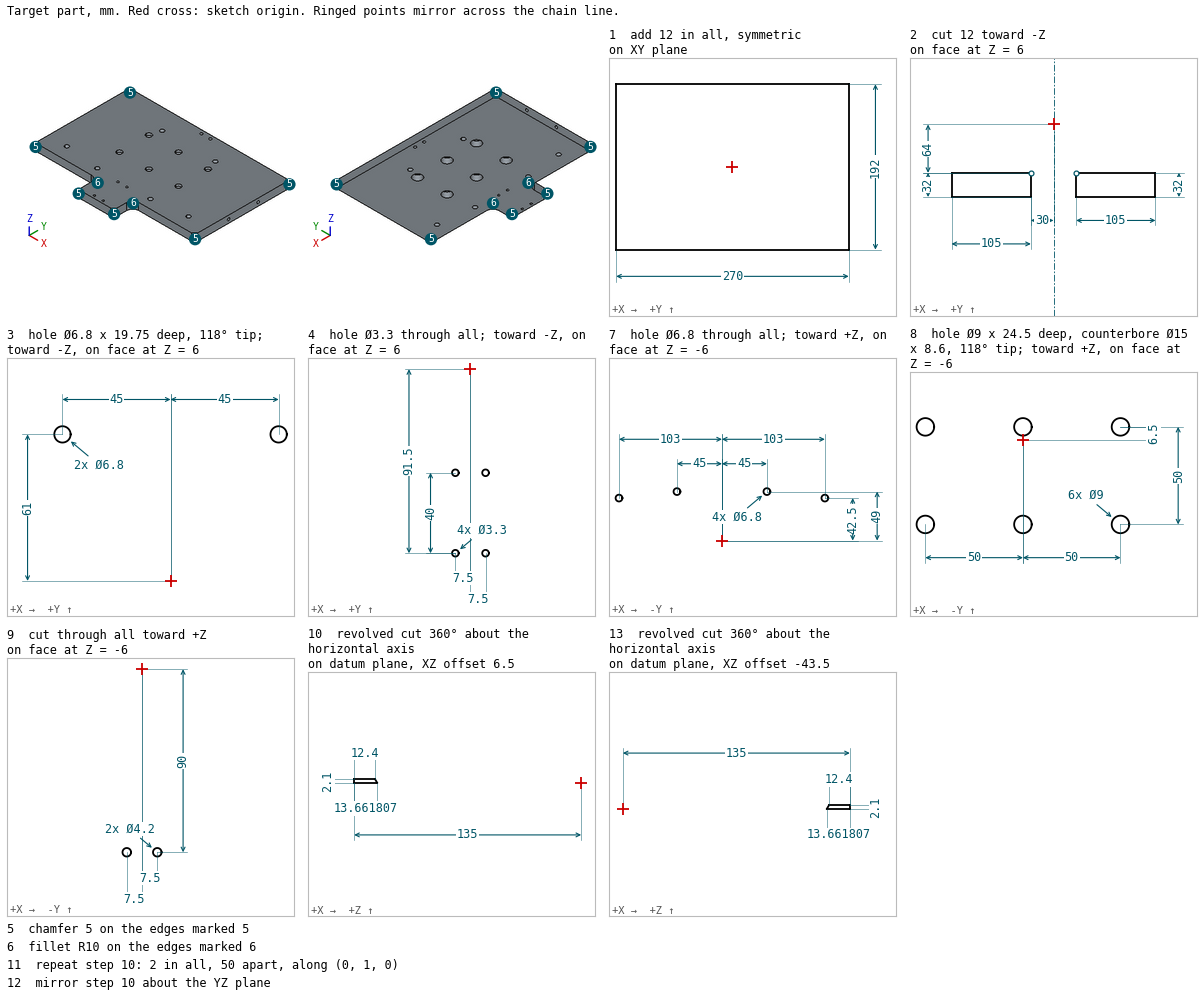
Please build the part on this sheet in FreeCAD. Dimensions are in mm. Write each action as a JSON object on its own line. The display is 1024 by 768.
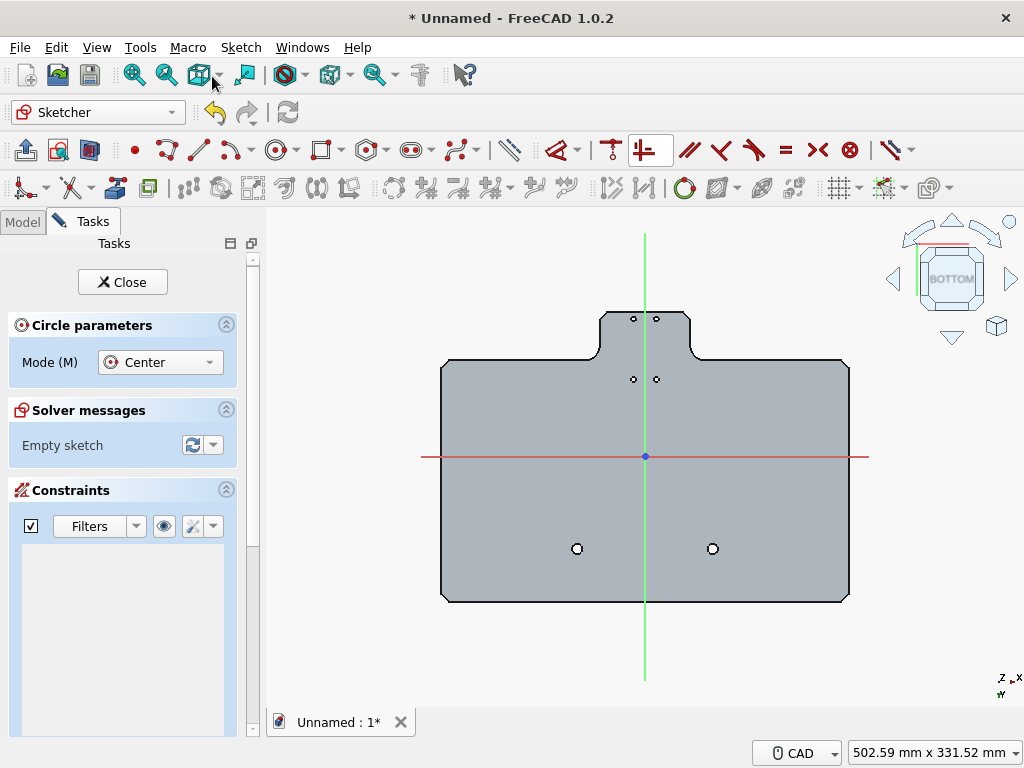
{"action": "scroll", "coordinate": [713, 383], "scroll_direction": "up", "scroll_amount": 8}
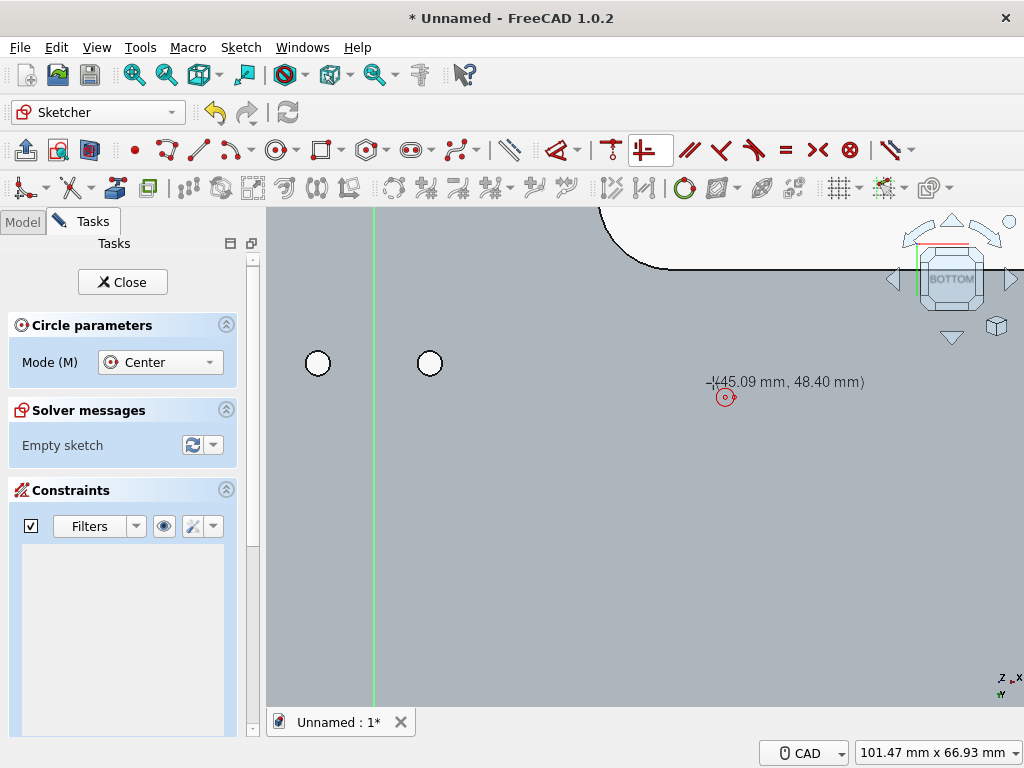
{"action": "scroll", "coordinate": [643, 426], "scroll_direction": "down", "scroll_amount": 7}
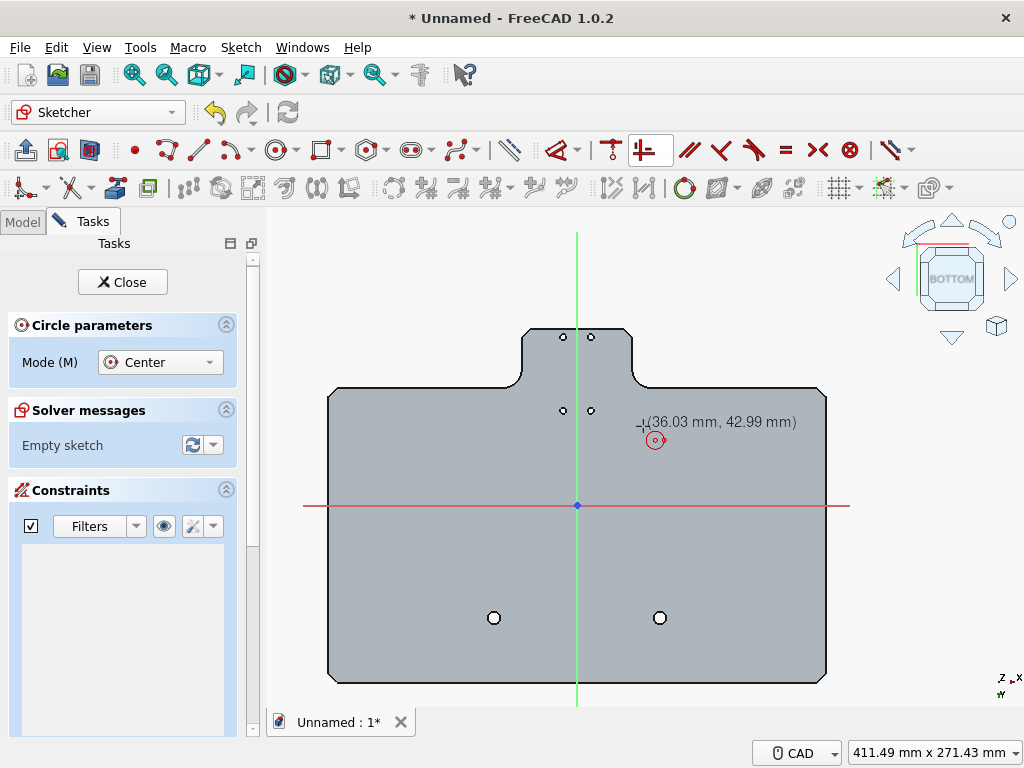
{"action": "left_click", "coordinate": [660, 416]}
{"action": "mouse_move", "coordinate": [664, 411]}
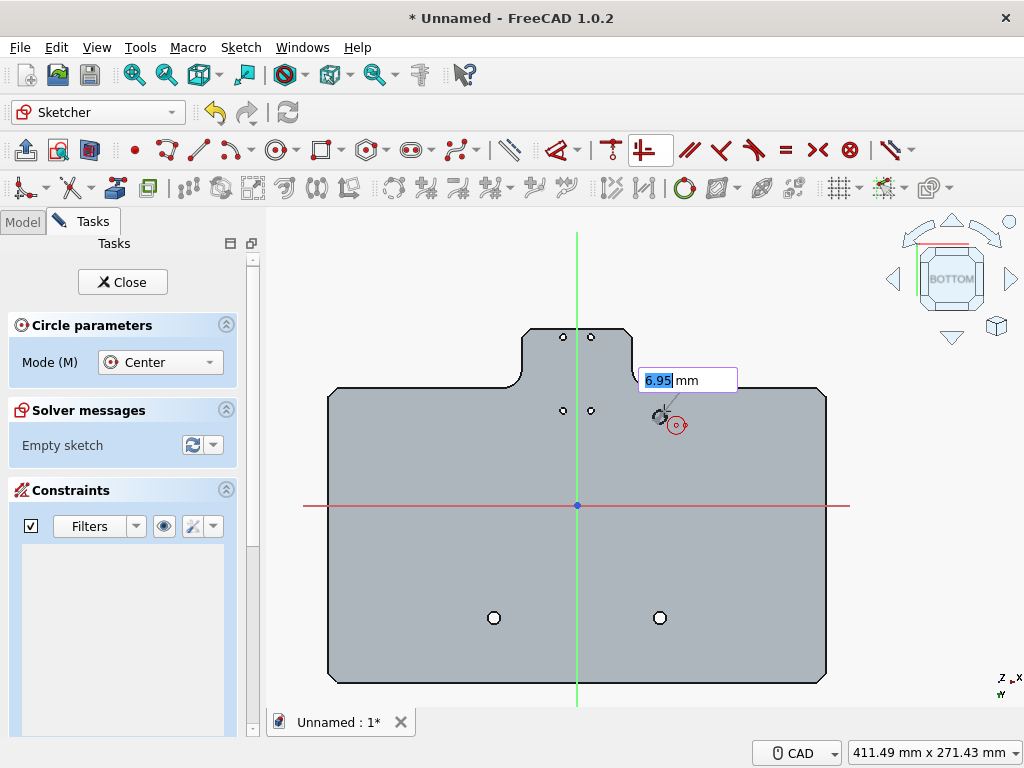
{"action": "type", "text": "6.8"}
{"action": "key", "text": "Return"}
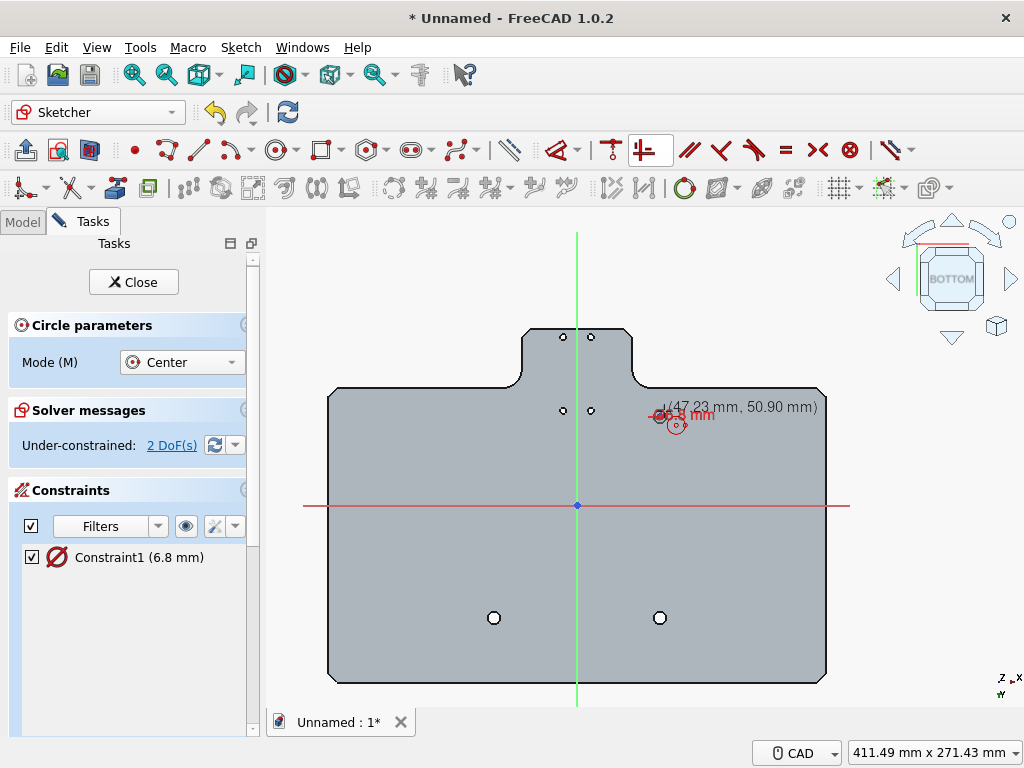
{"action": "scroll", "coordinate": [494, 416], "scroll_direction": "up", "scroll_amount": 7}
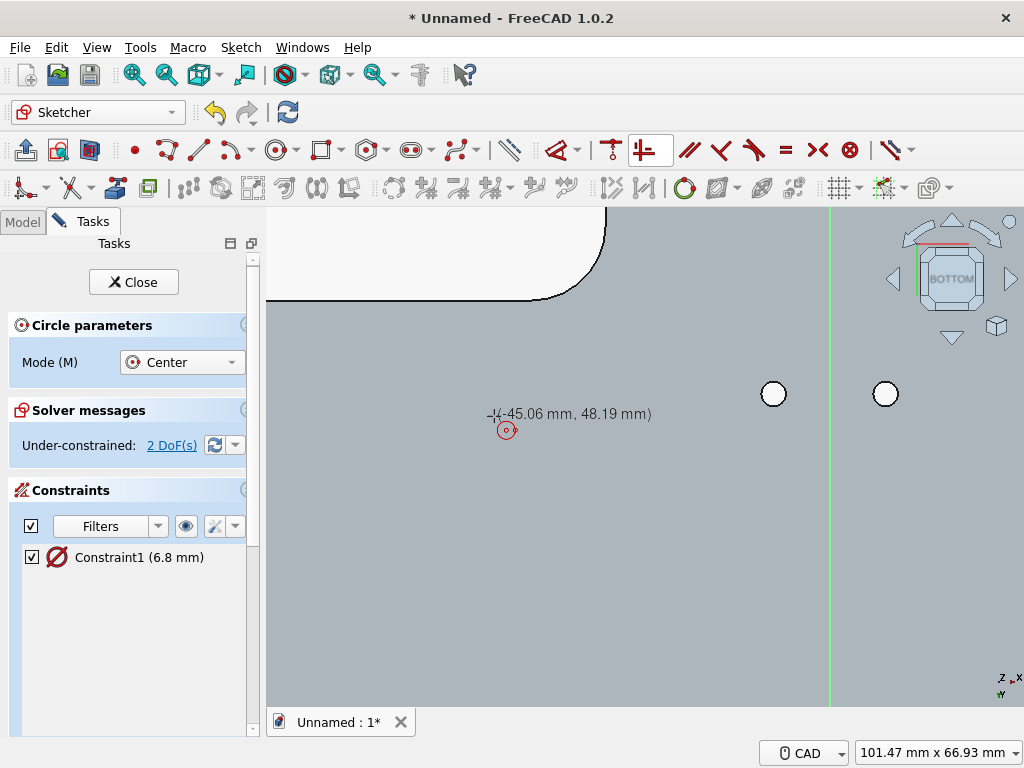
{"action": "scroll", "coordinate": [494, 416], "scroll_direction": "down", "scroll_amount": 7}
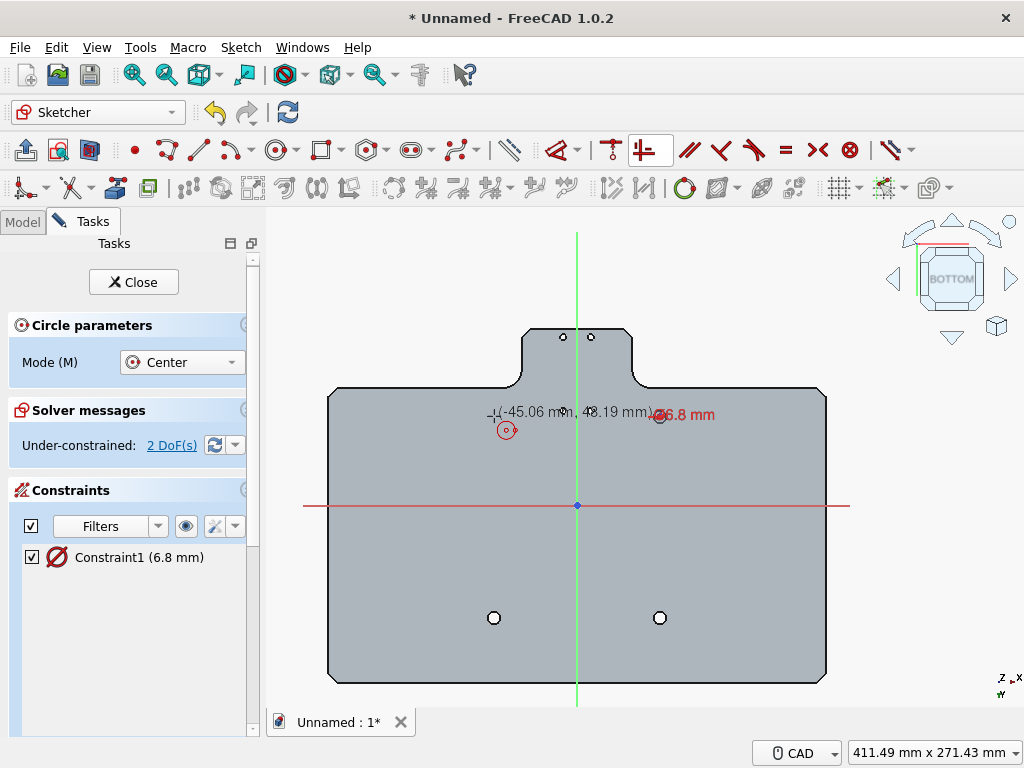
{"action": "left_click", "coordinate": [494, 416]}
{"action": "mouse_move", "coordinate": [499, 411]}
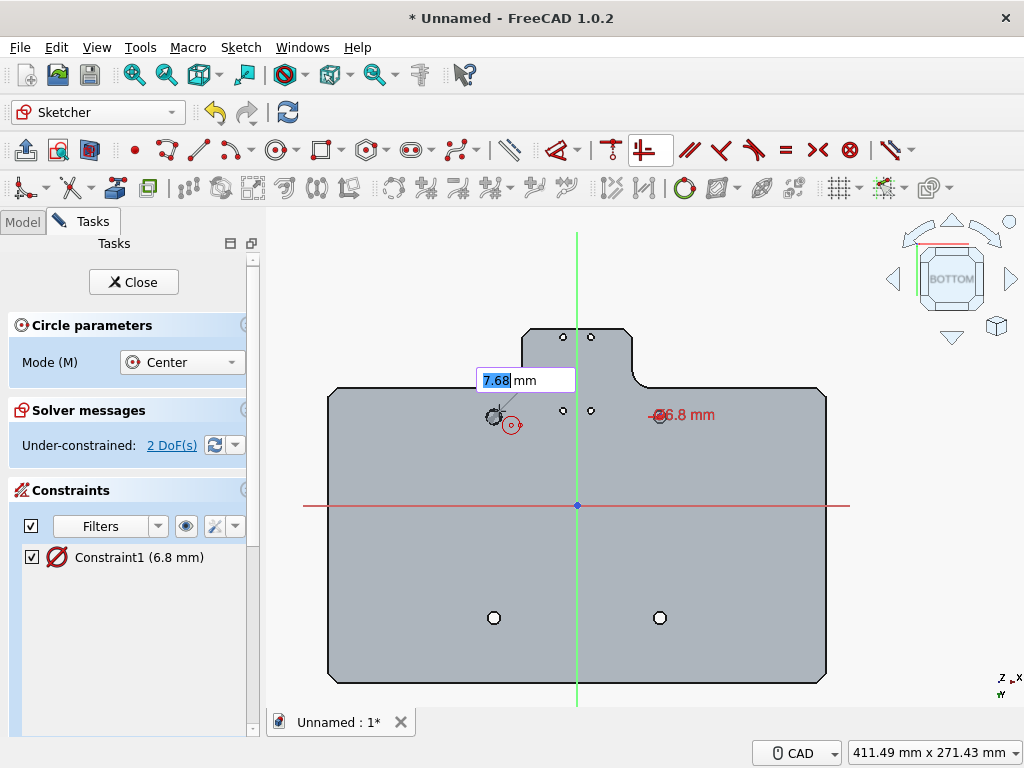
{"action": "type", "text": "6.8"}
{"action": "key", "text": "Return"}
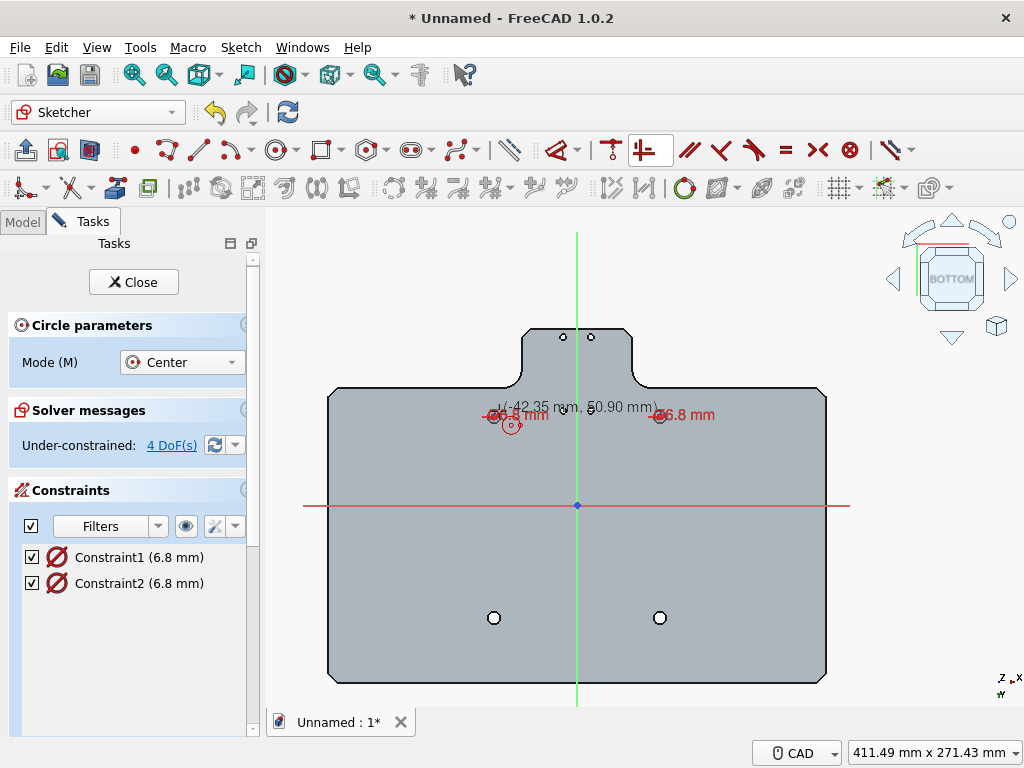
{"action": "scroll", "coordinate": [767, 427], "scroll_direction": "up", "scroll_amount": 7}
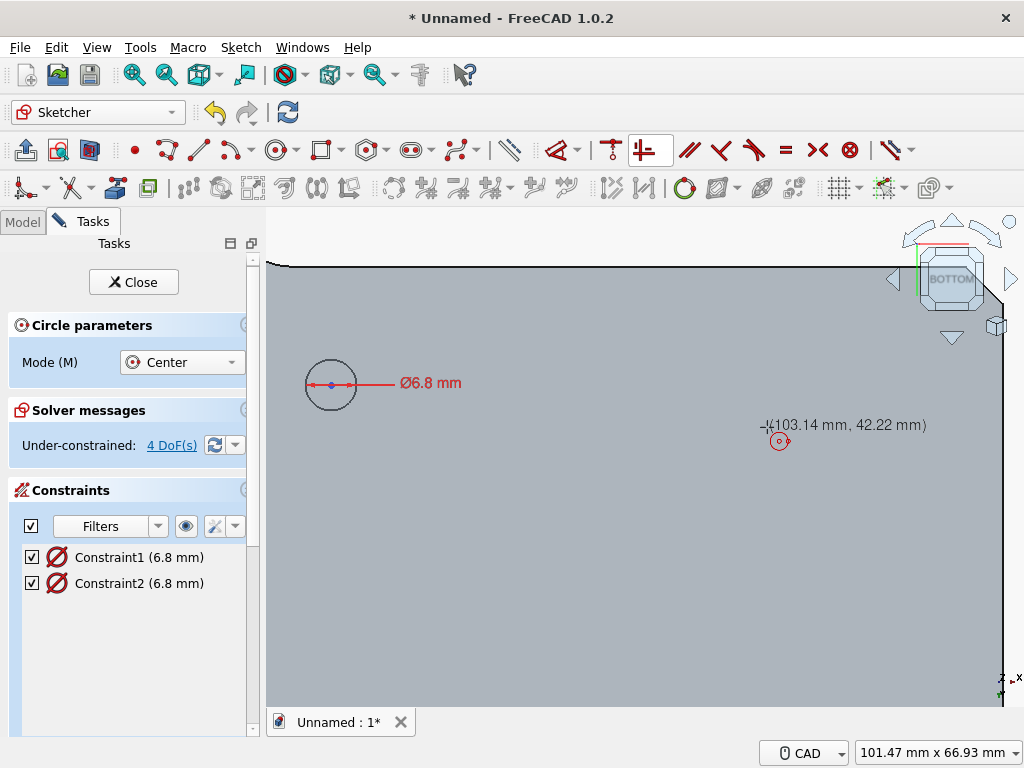
{"action": "scroll", "coordinate": [767, 427], "scroll_direction": "down", "scroll_amount": 7}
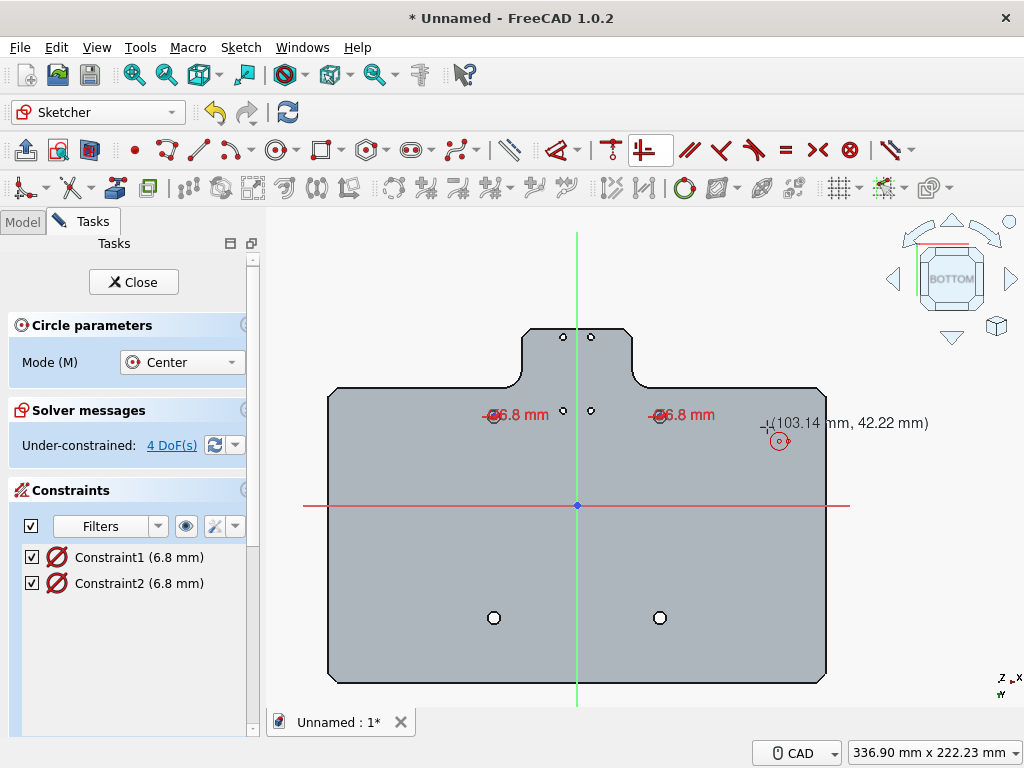
{"action": "left_click", "coordinate": [767, 427]}
{"action": "mouse_move", "coordinate": [771, 423]}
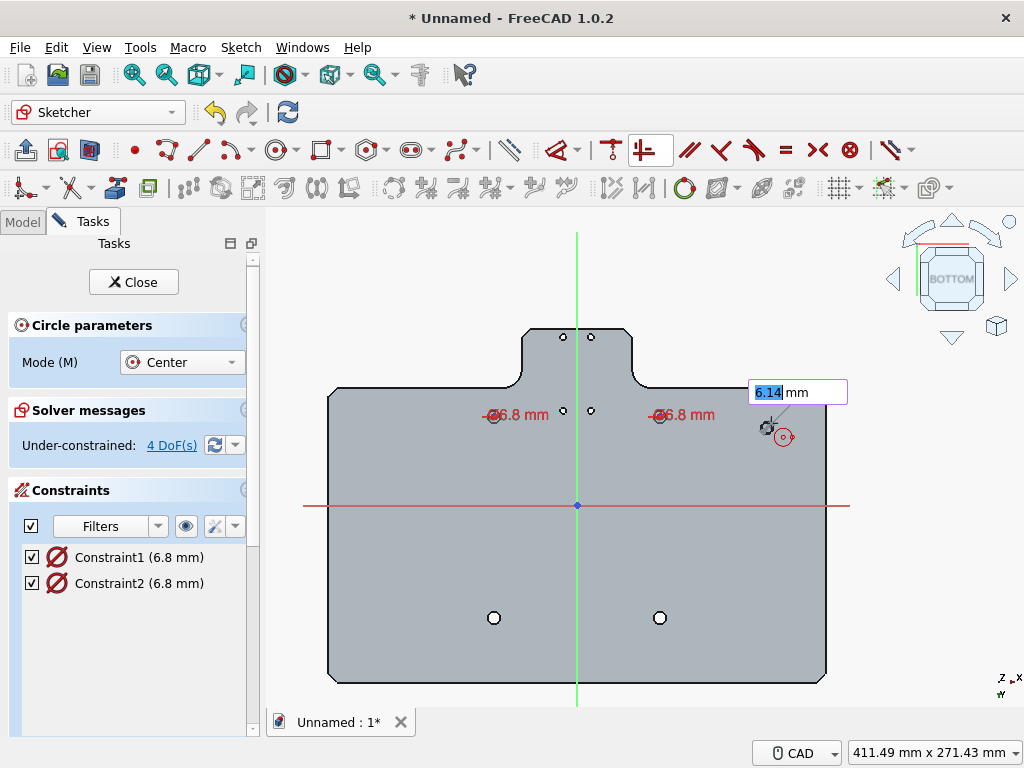
{"action": "type", "text": "6.8"}
{"action": "key", "text": "Return"}